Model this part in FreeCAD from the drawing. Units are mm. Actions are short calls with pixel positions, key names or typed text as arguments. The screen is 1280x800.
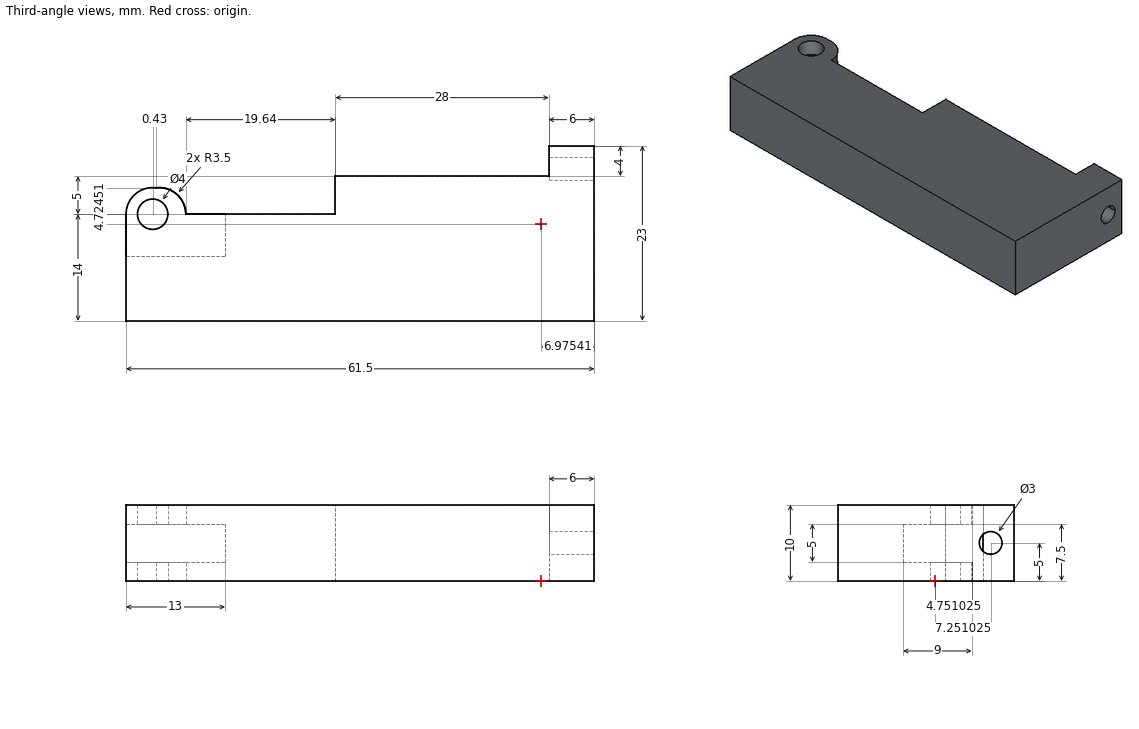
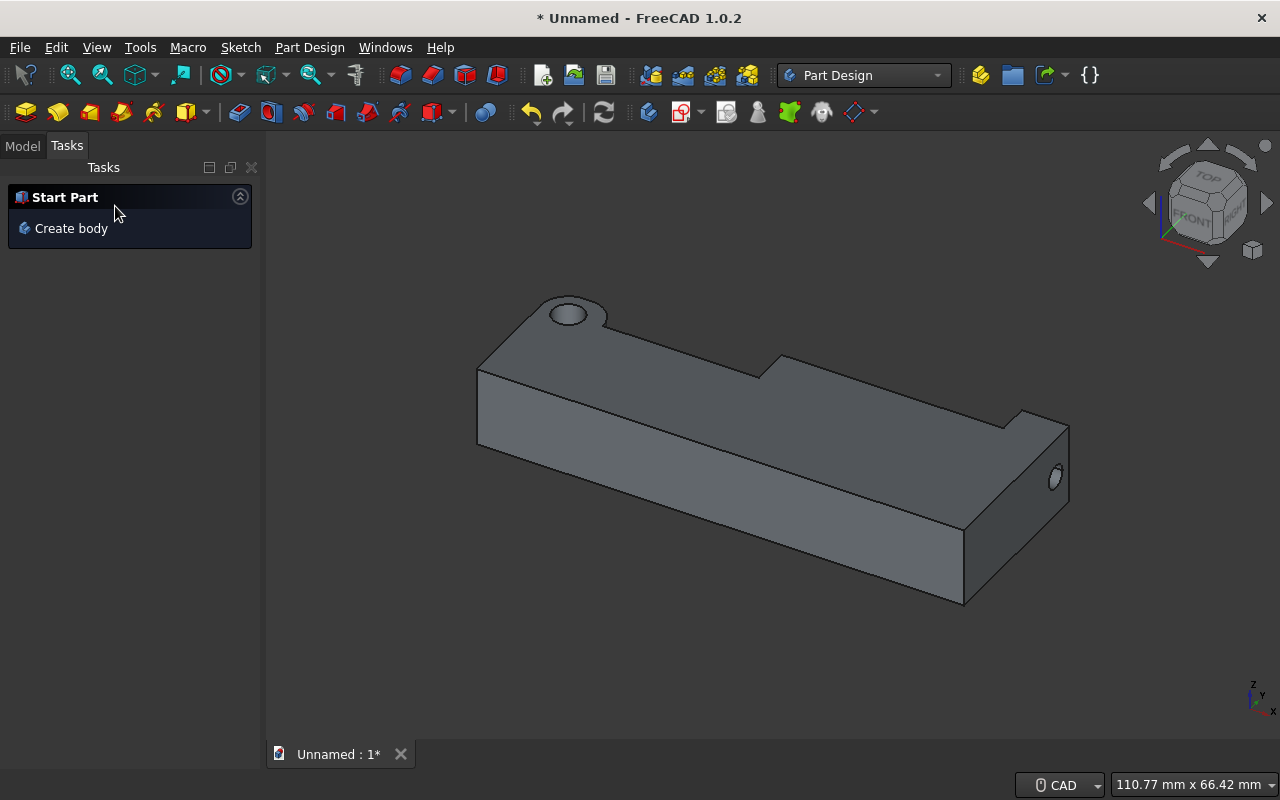
key(6)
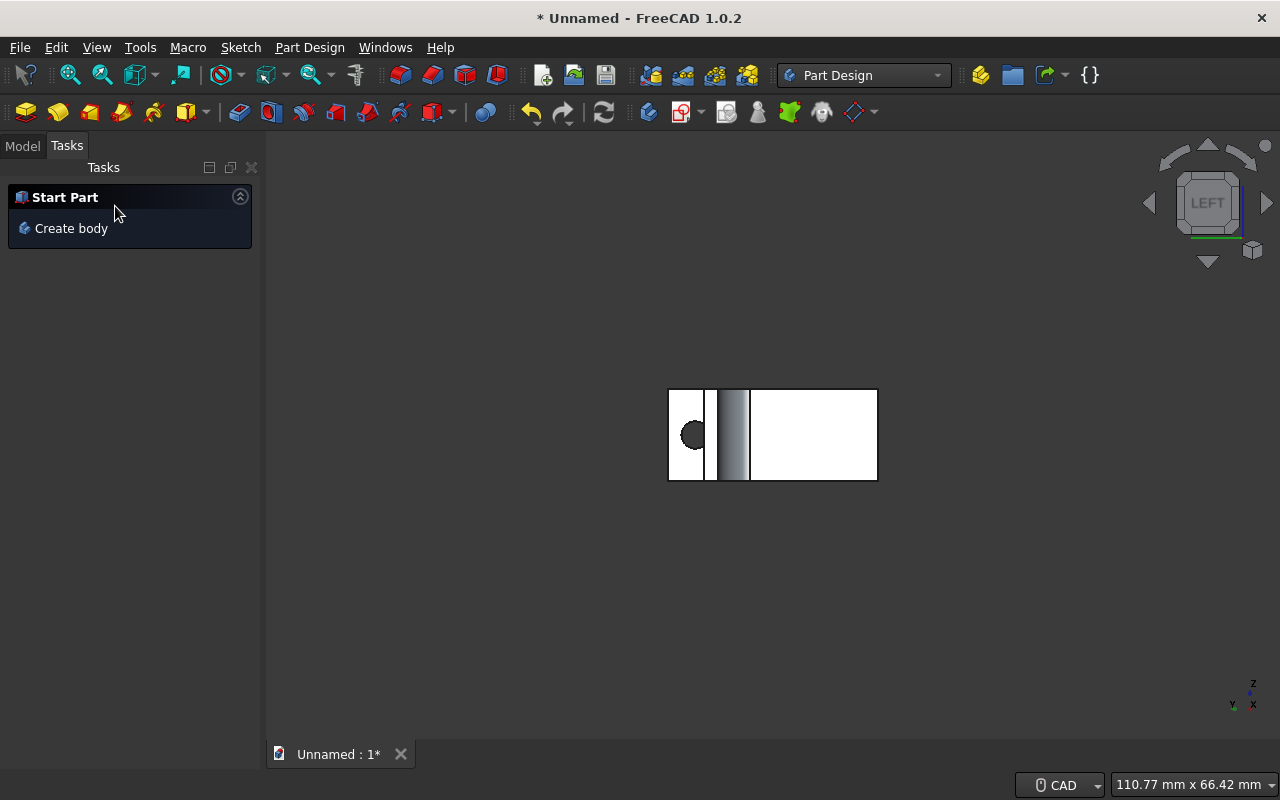
key(v)
key(f)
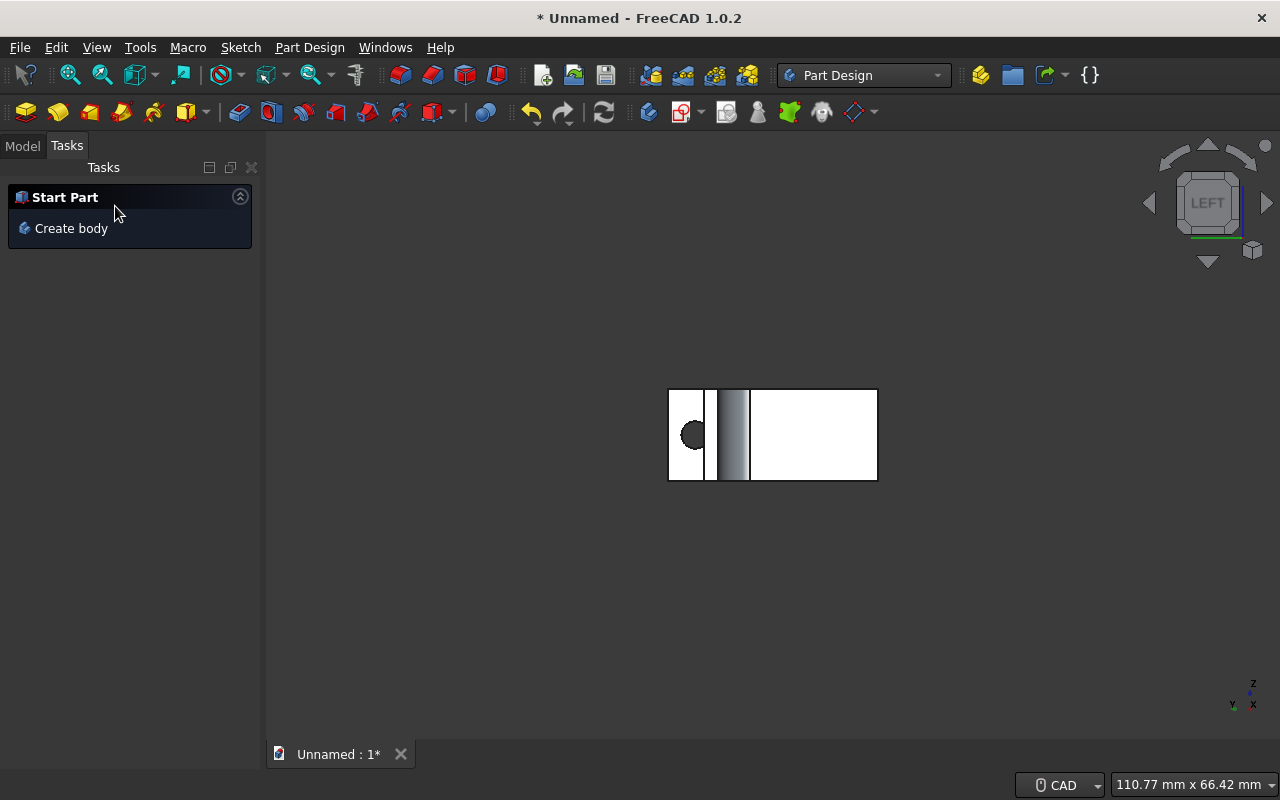
click(796, 434)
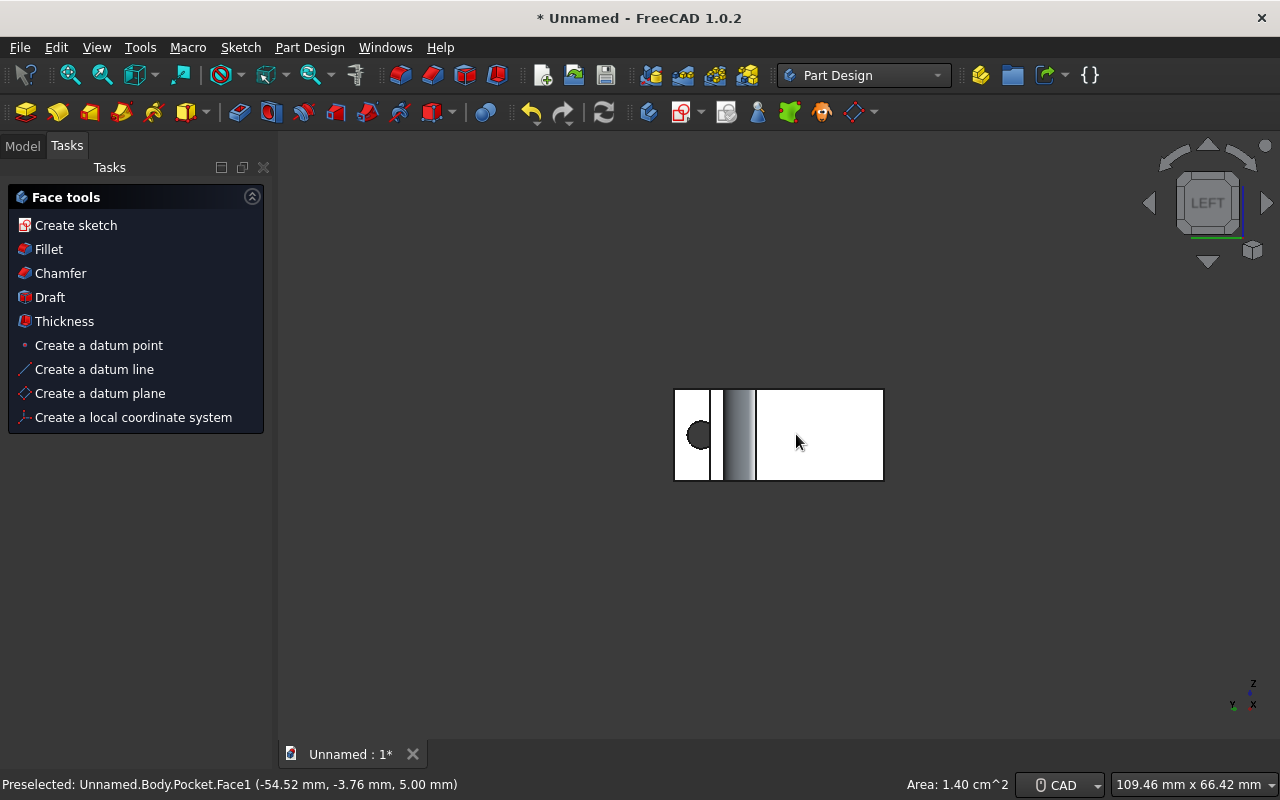
click(682, 112)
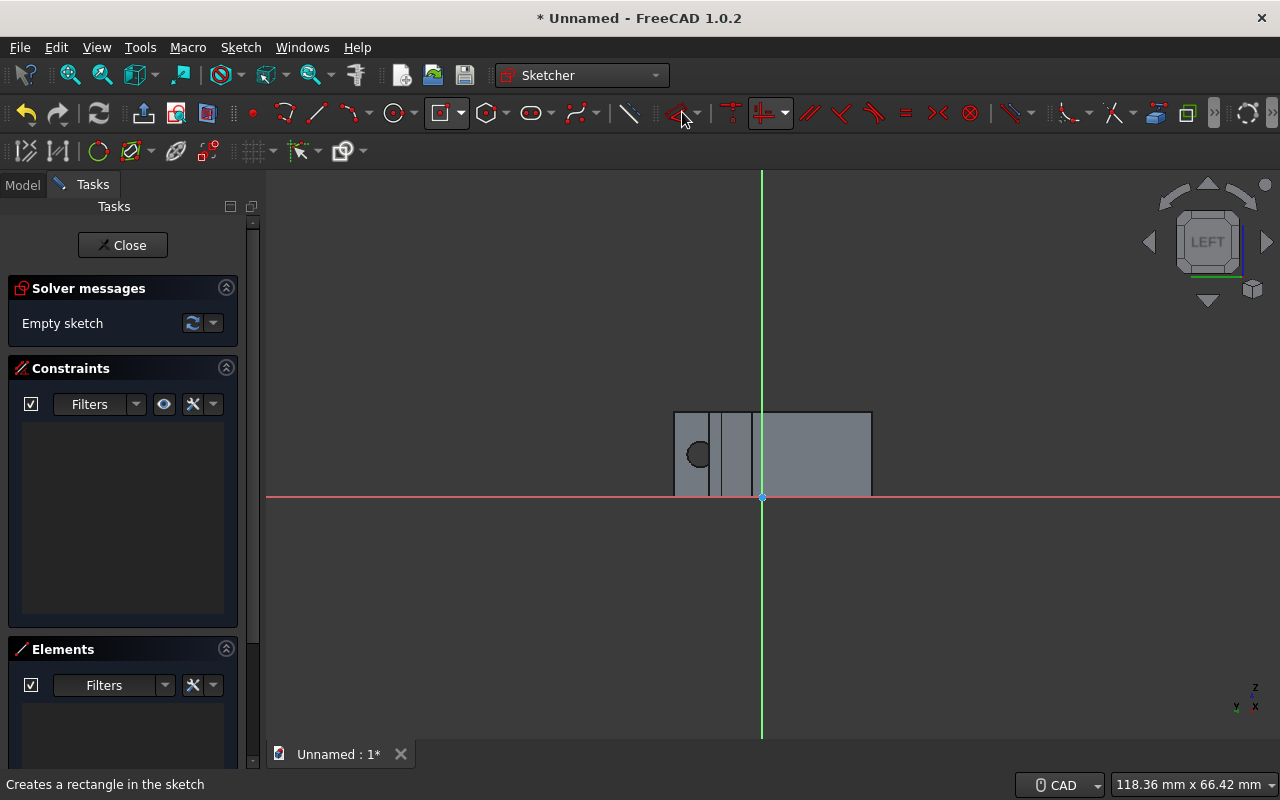
scroll(771, 467, up, 9)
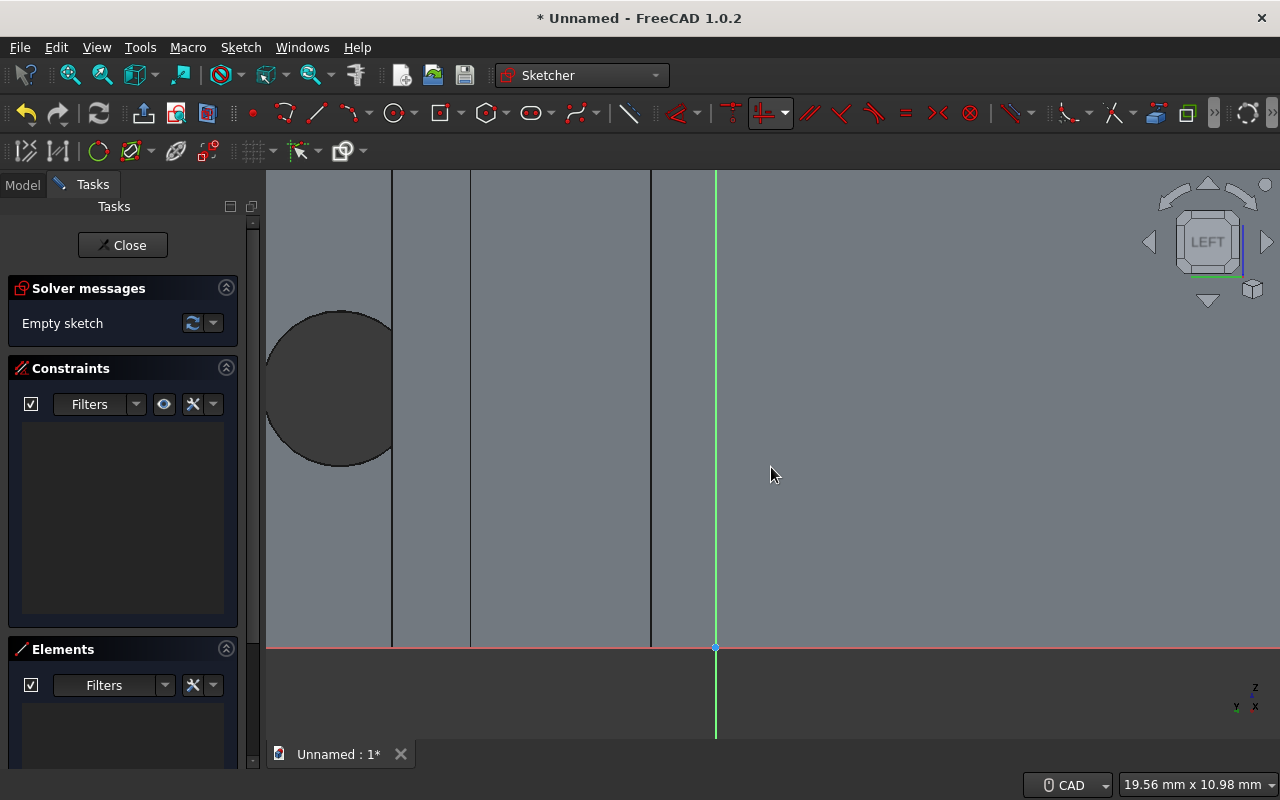
key(g)
key(r)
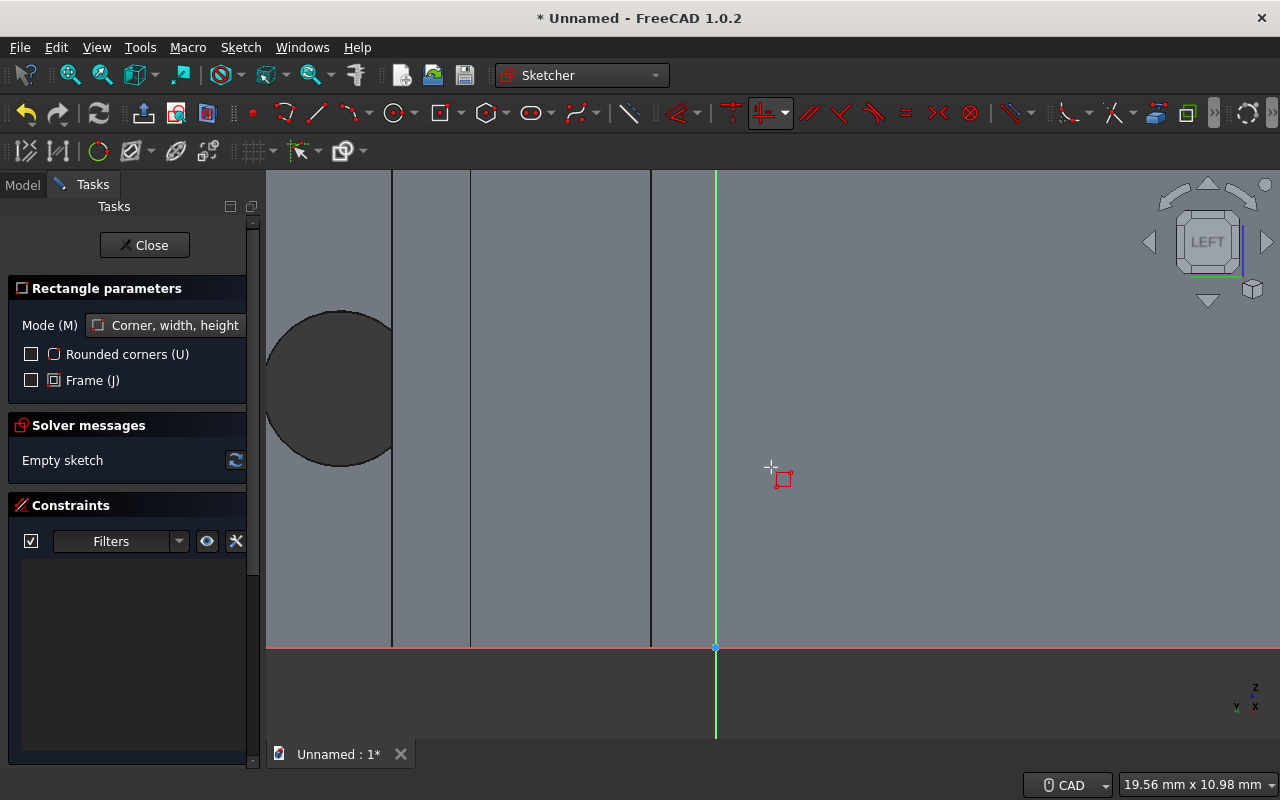
click(470, 259)
move(936, 518)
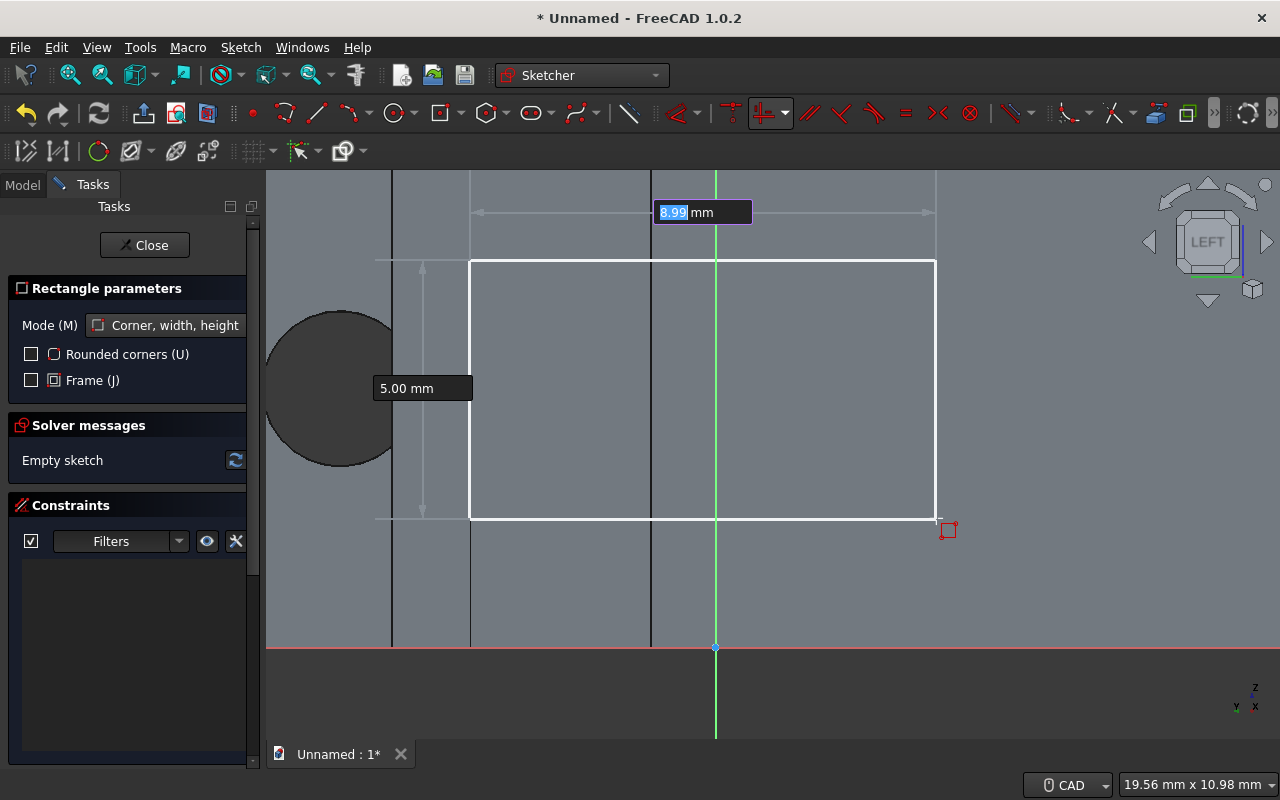
text(9)
key(Tab)
text(5)
key(Return)
key(Escape)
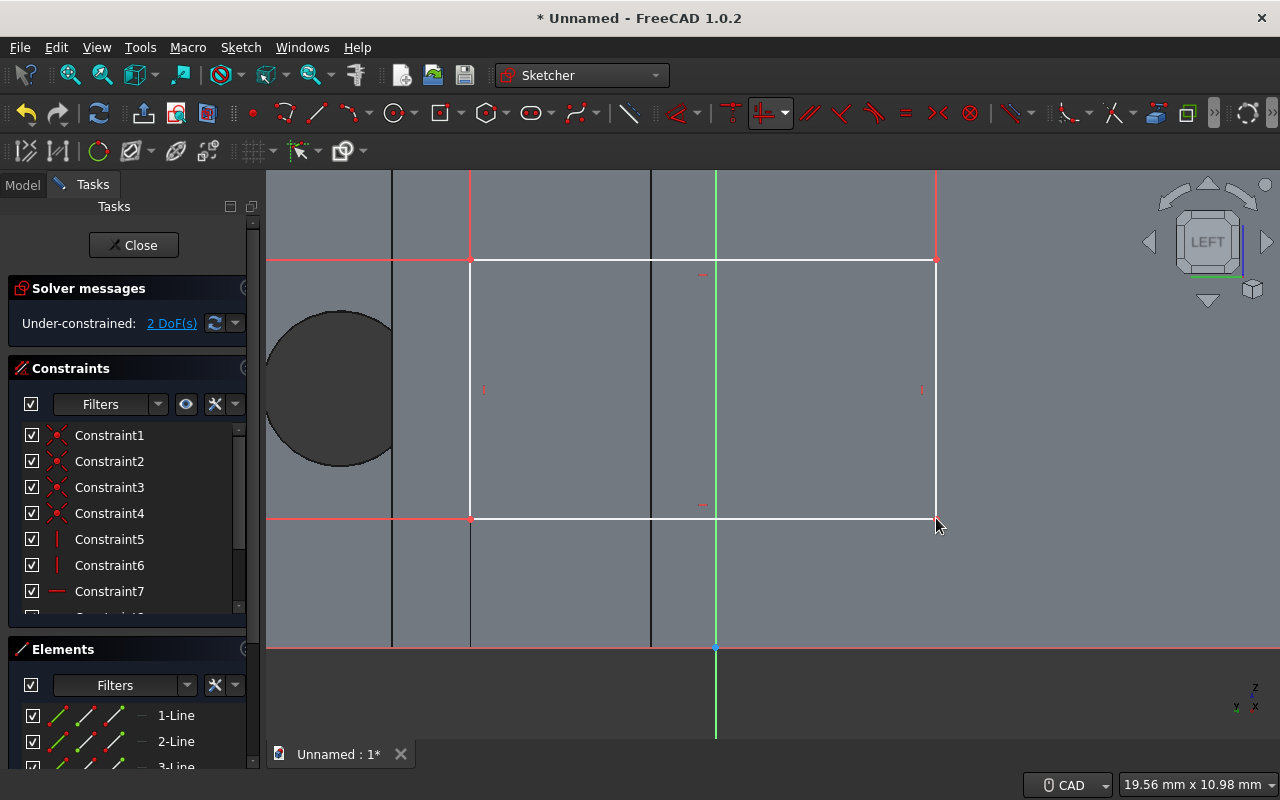
click(676, 114)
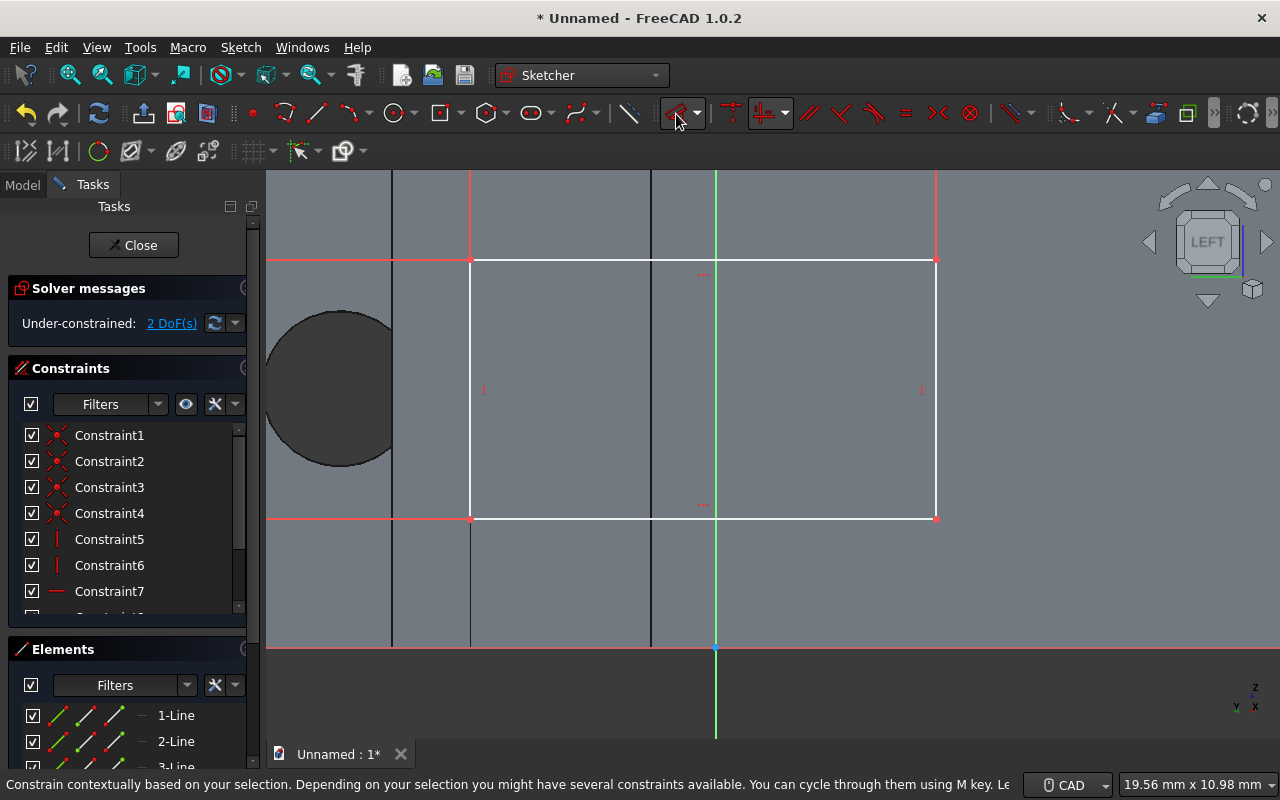
click(470, 260)
click(436, 454)